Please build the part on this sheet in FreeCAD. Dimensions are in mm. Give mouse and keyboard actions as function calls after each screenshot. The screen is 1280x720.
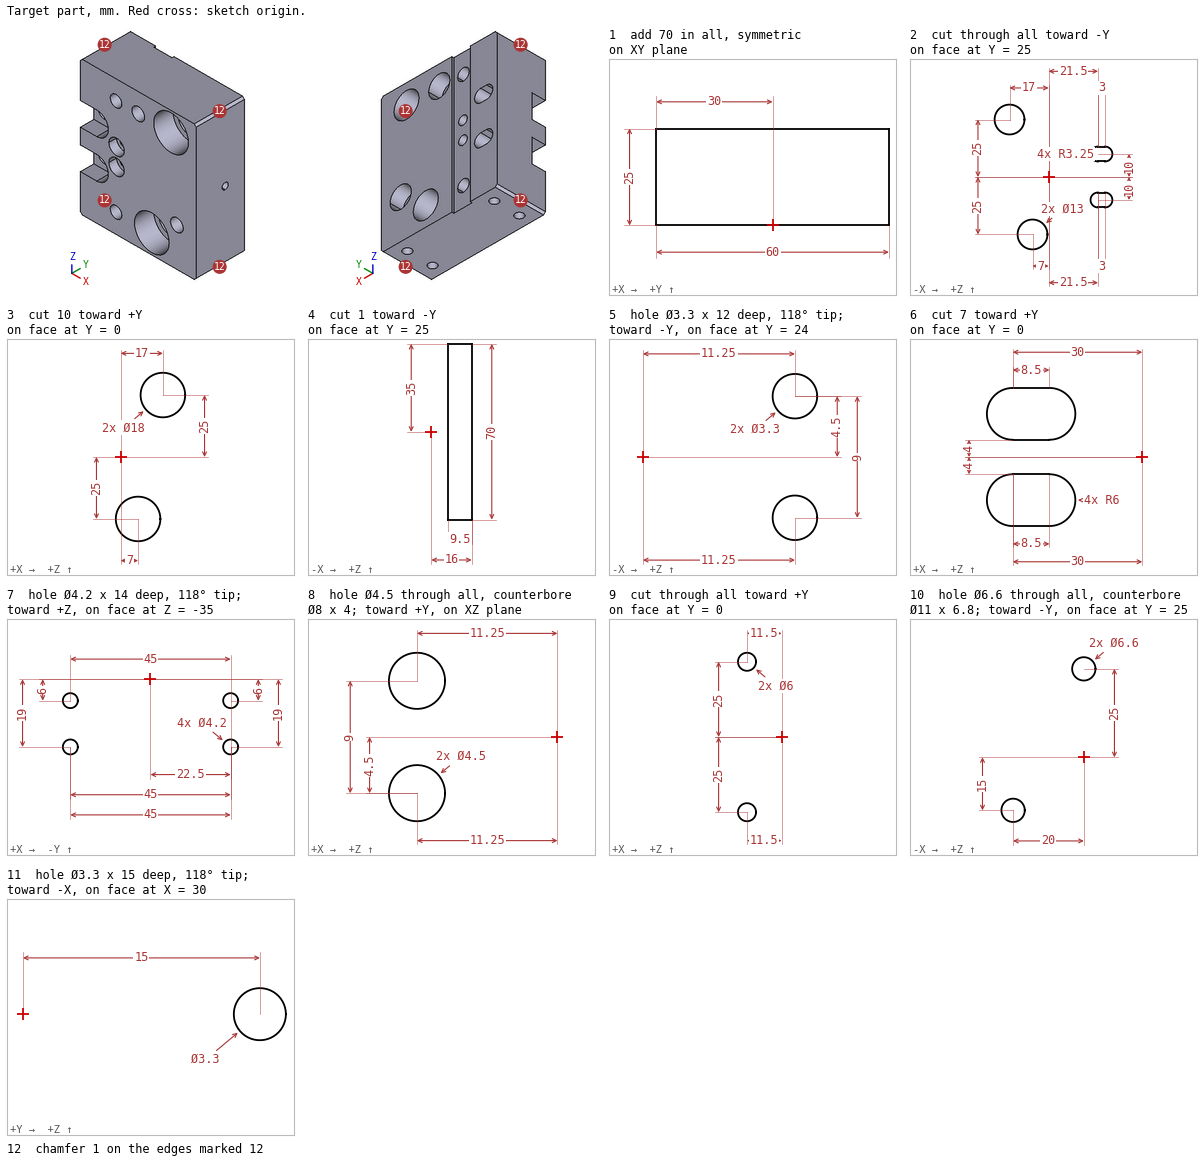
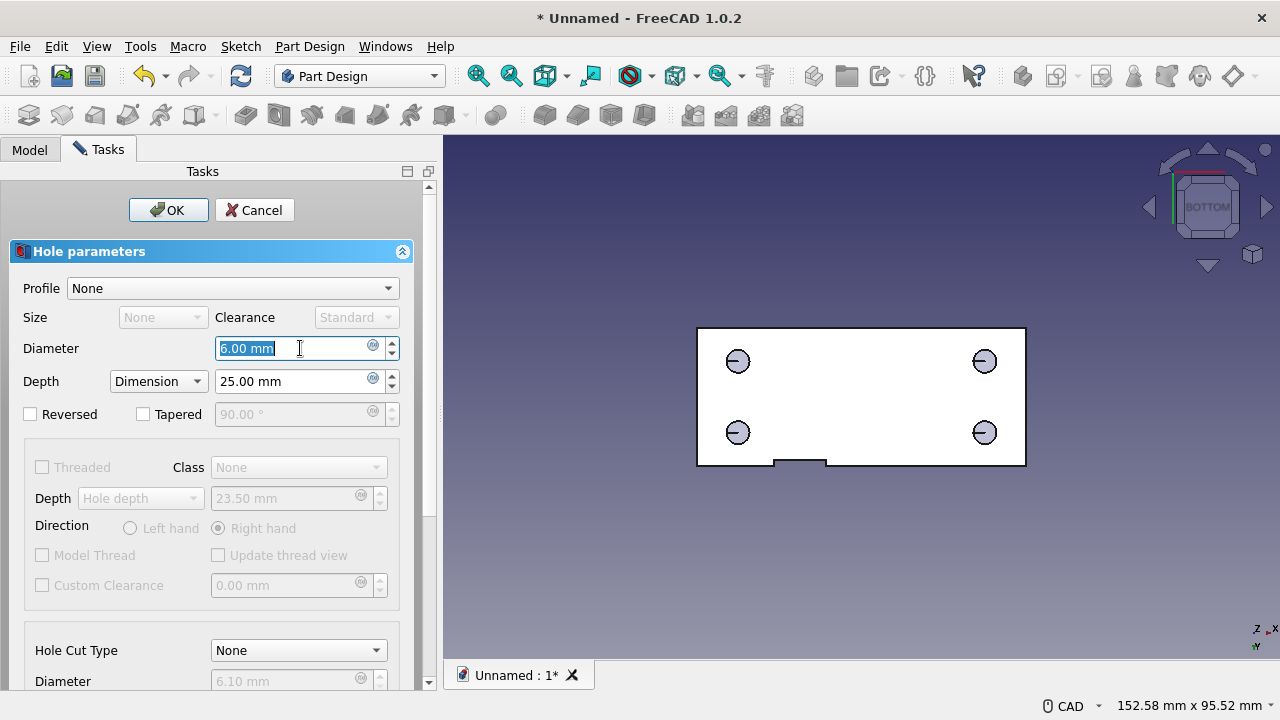
text(4.5)
key(Tab)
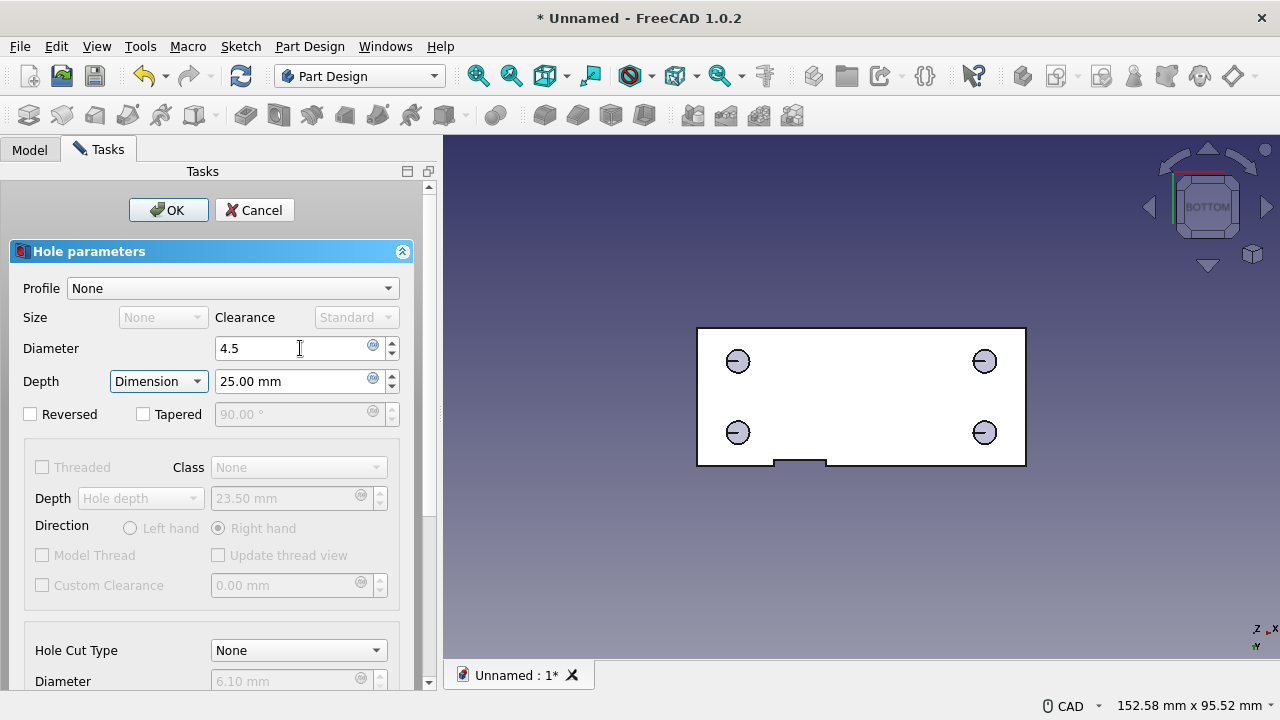
click(160, 382)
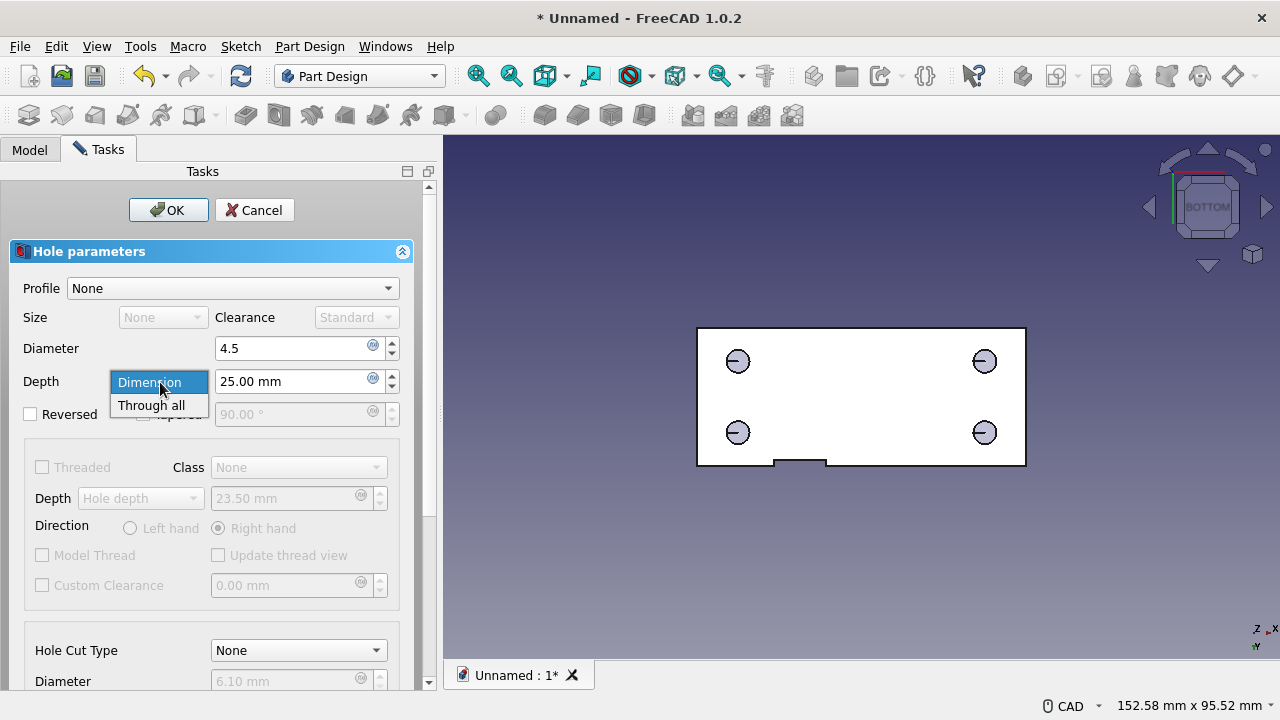
click(158, 406)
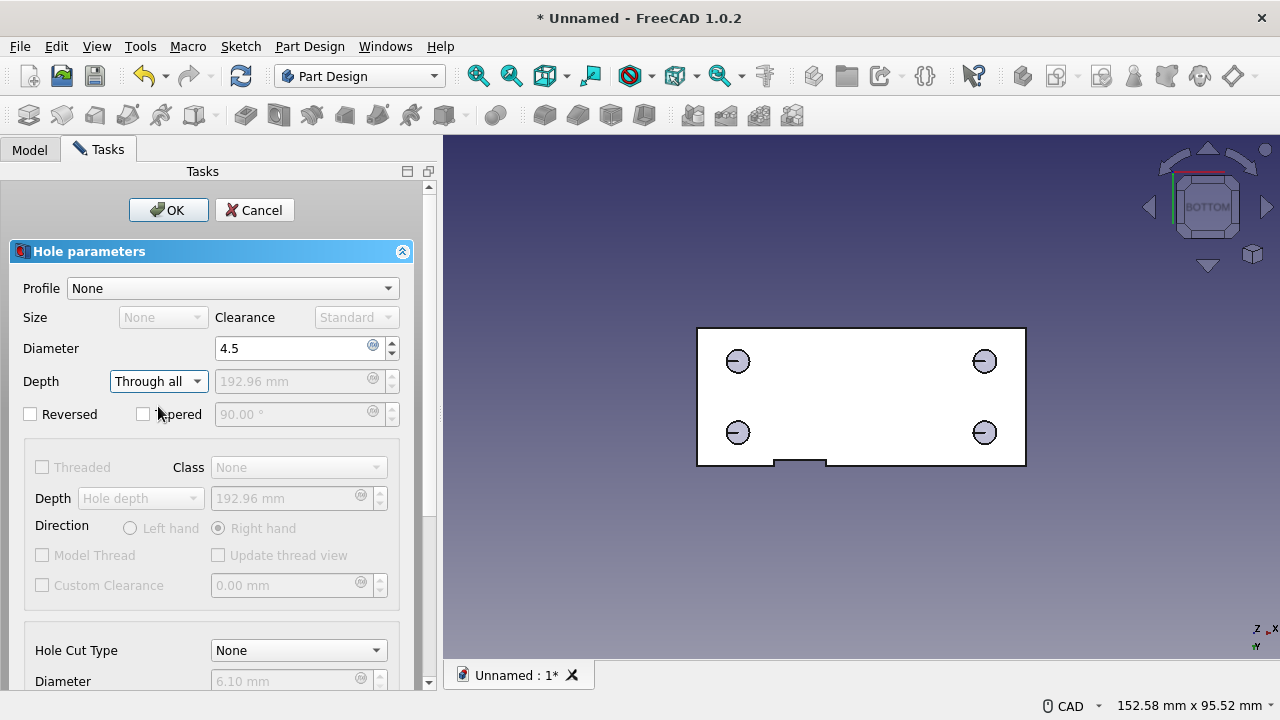
click(300, 650)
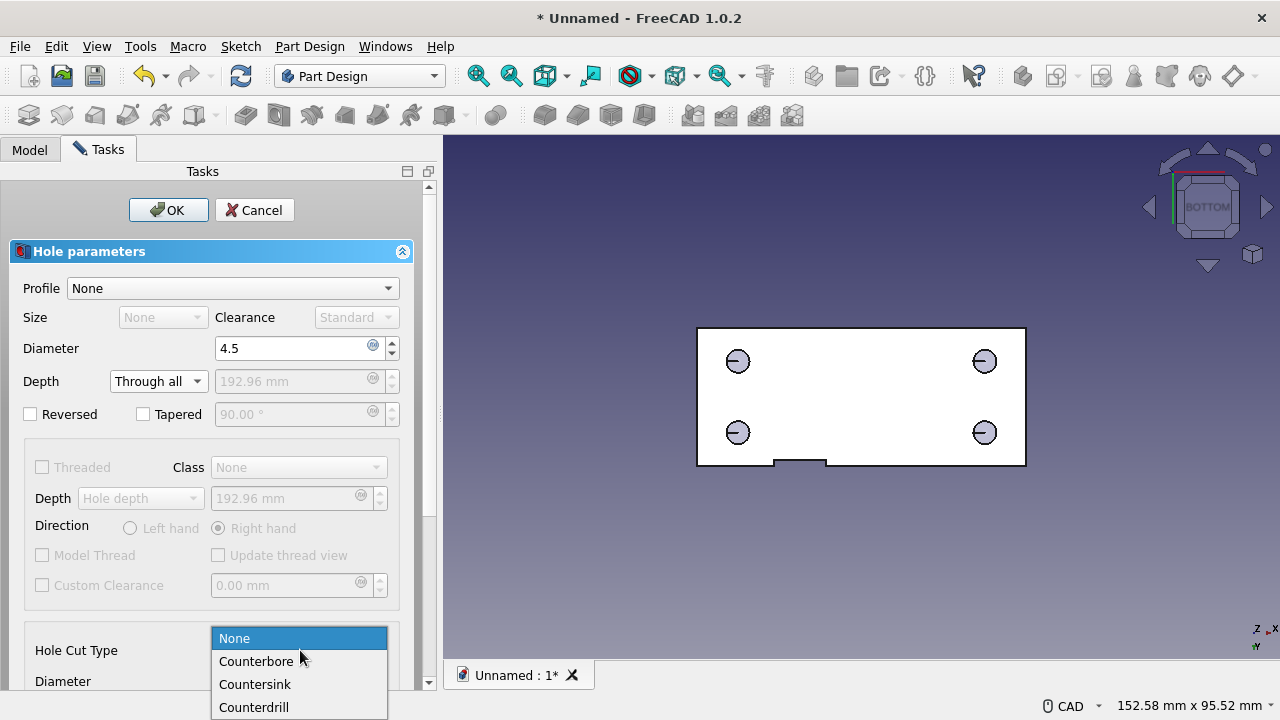
click(298, 662)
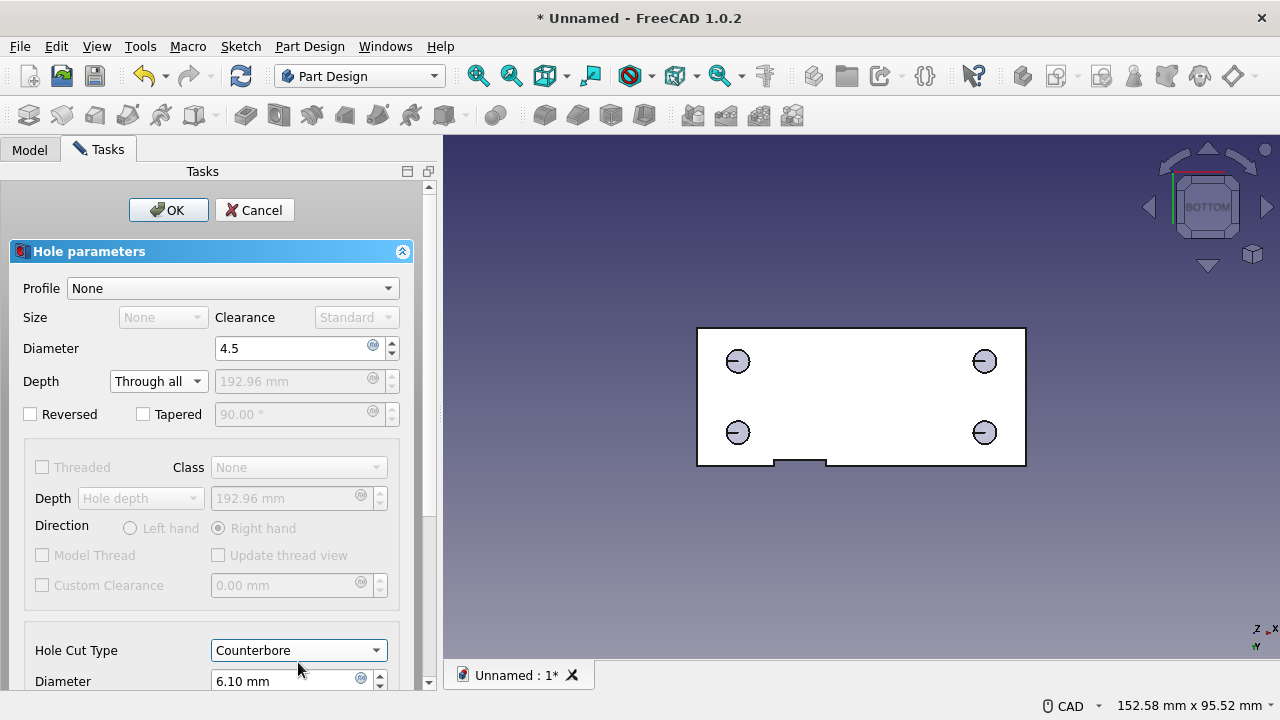
scroll(429, 436, down, 2)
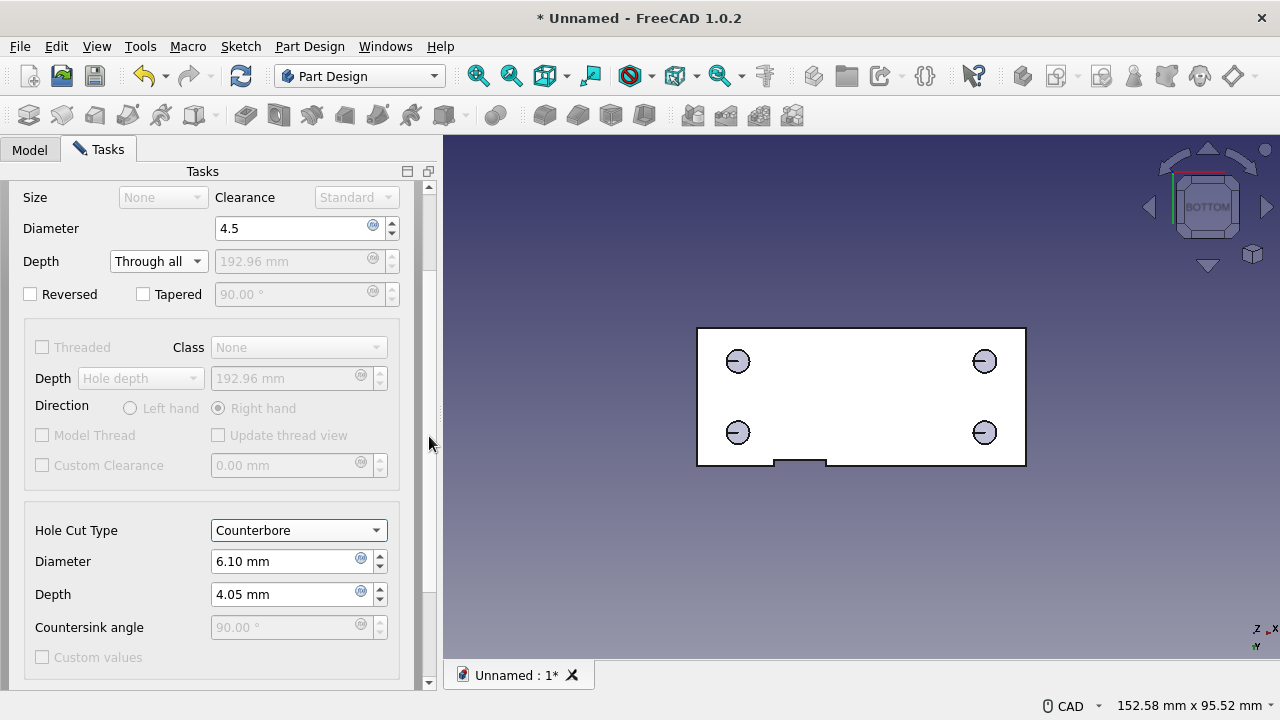
triple_click(292, 562)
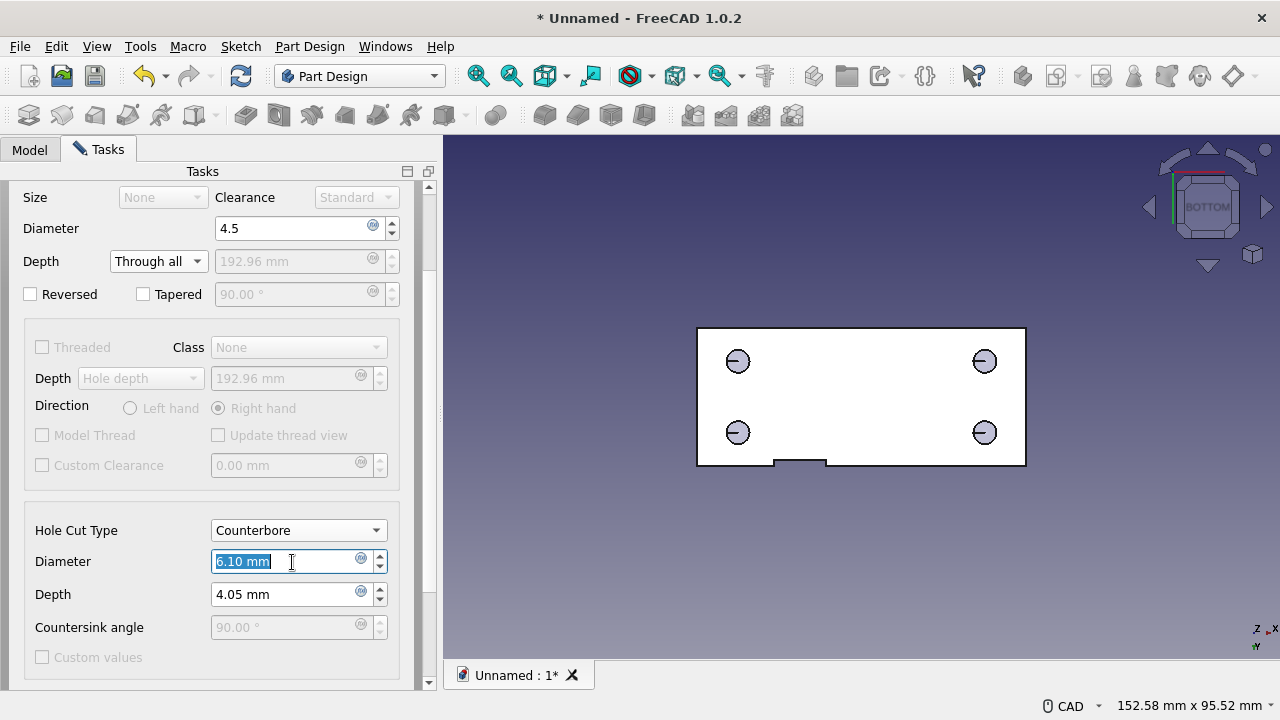
text(8)
key(Tab)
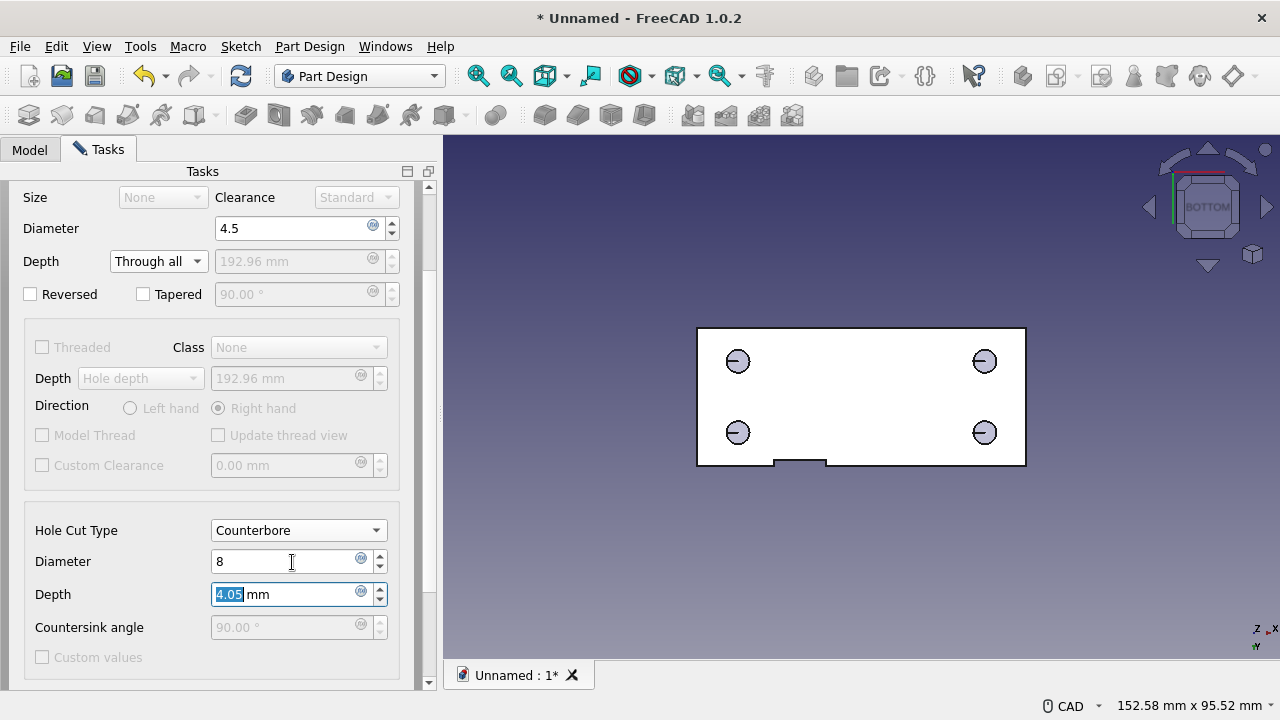
text(4)
key(Tab)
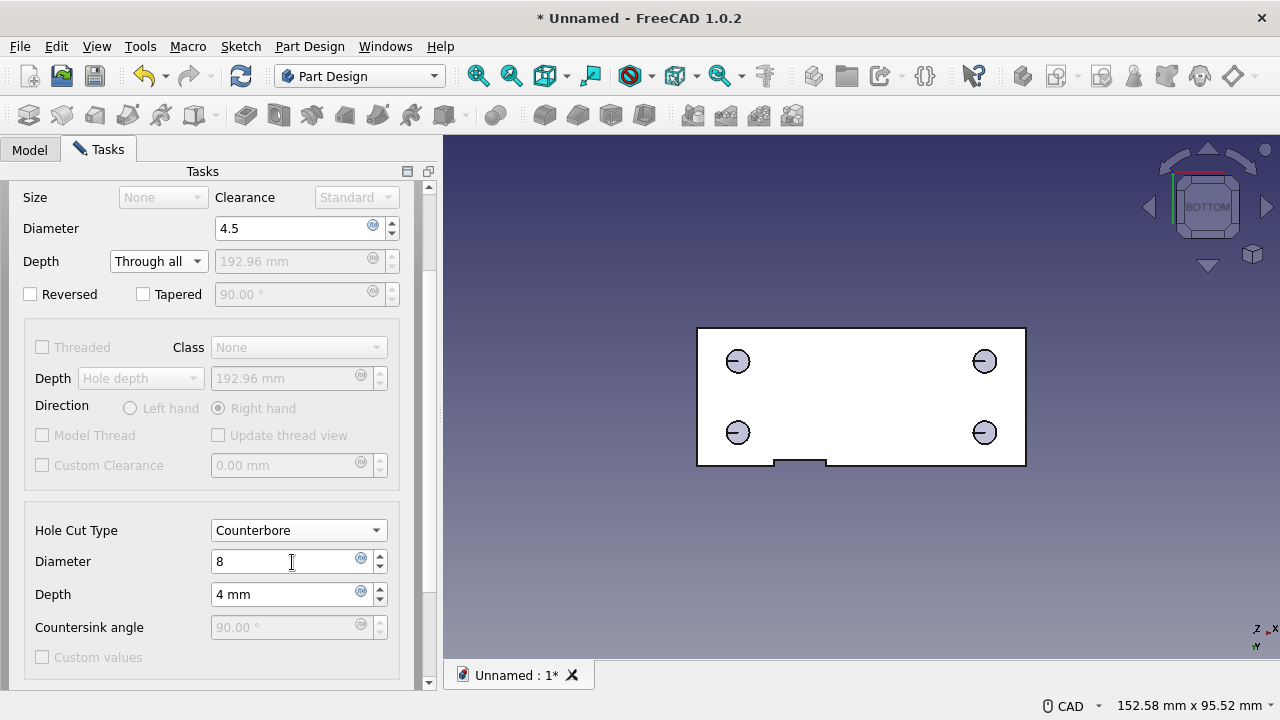
scroll(429, 436, up, 3)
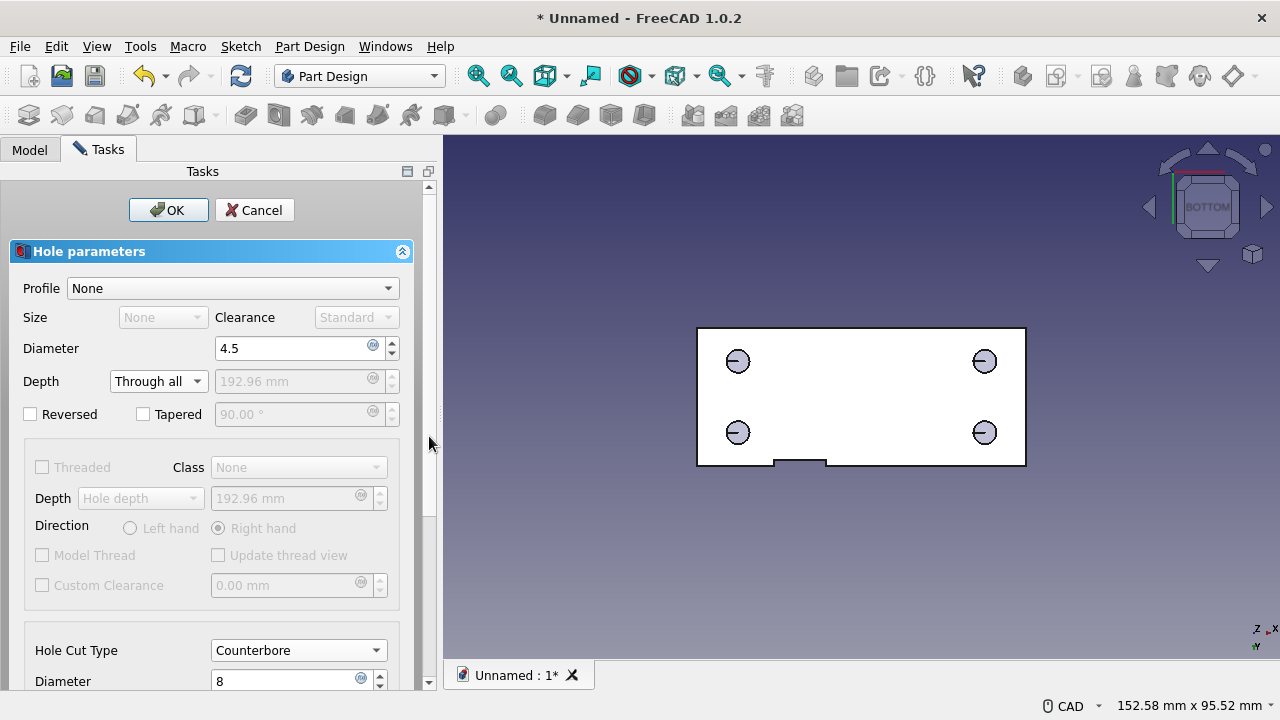
click(169, 210)